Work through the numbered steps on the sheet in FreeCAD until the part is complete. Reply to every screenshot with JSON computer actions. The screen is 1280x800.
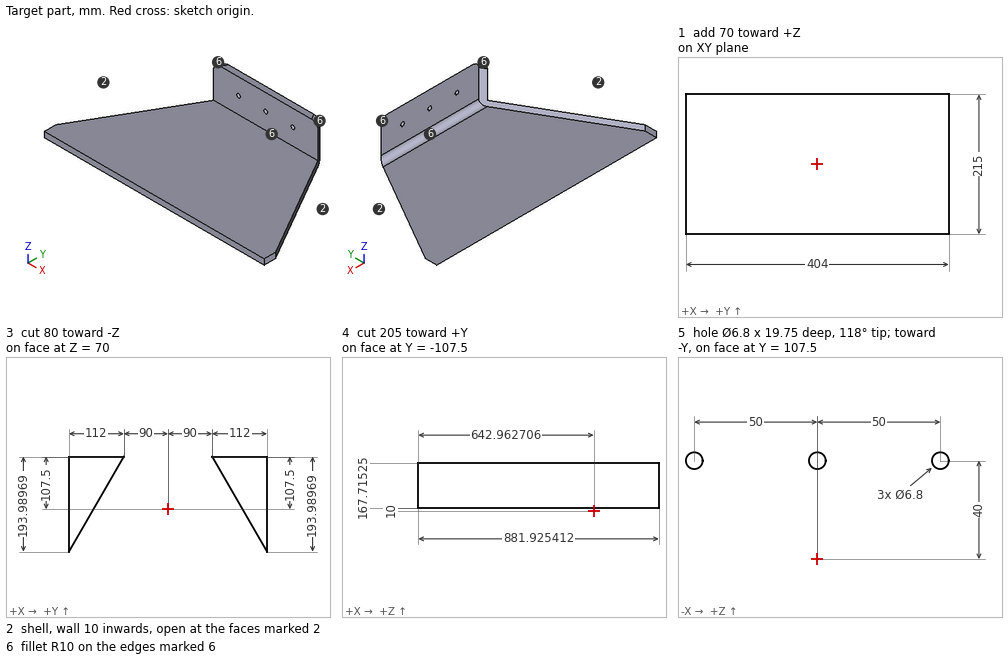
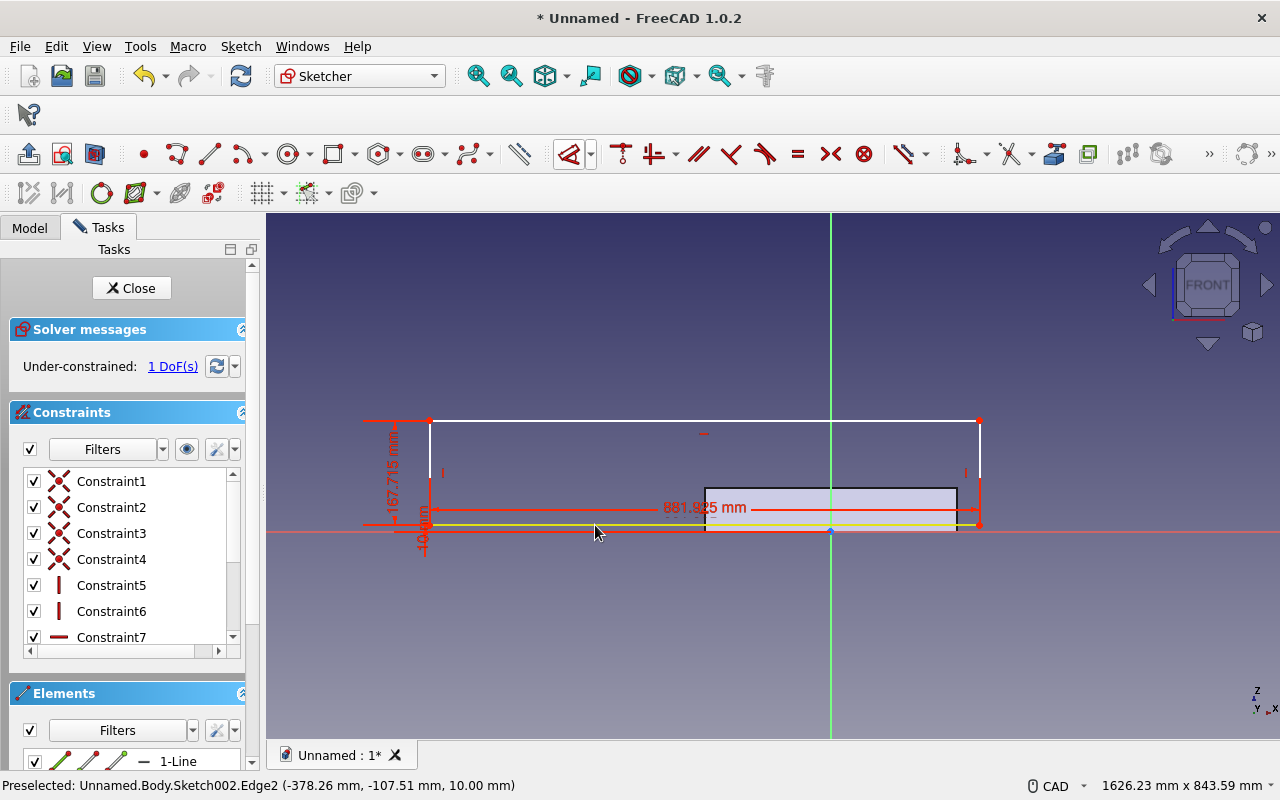
{"action": "left_click", "coordinate": [430, 421]}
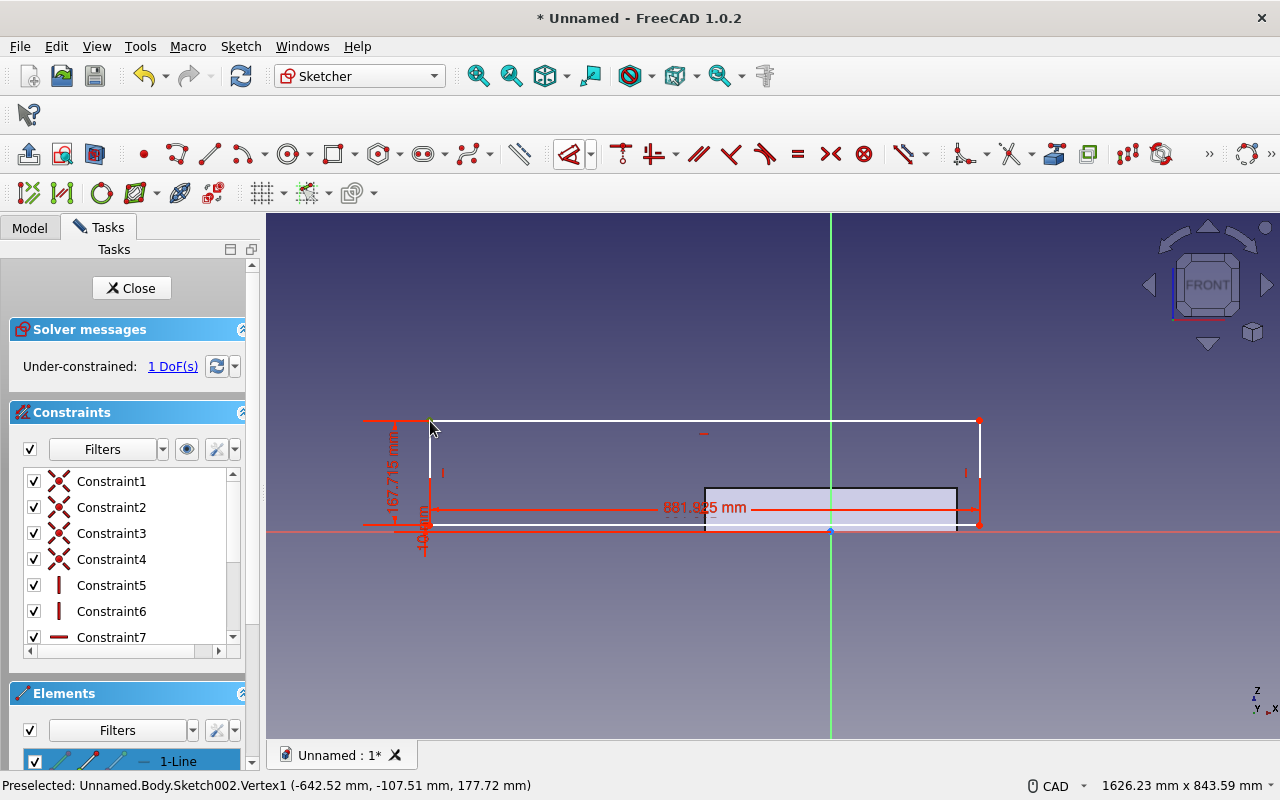
{"action": "left_click", "coordinate": [590, 154]}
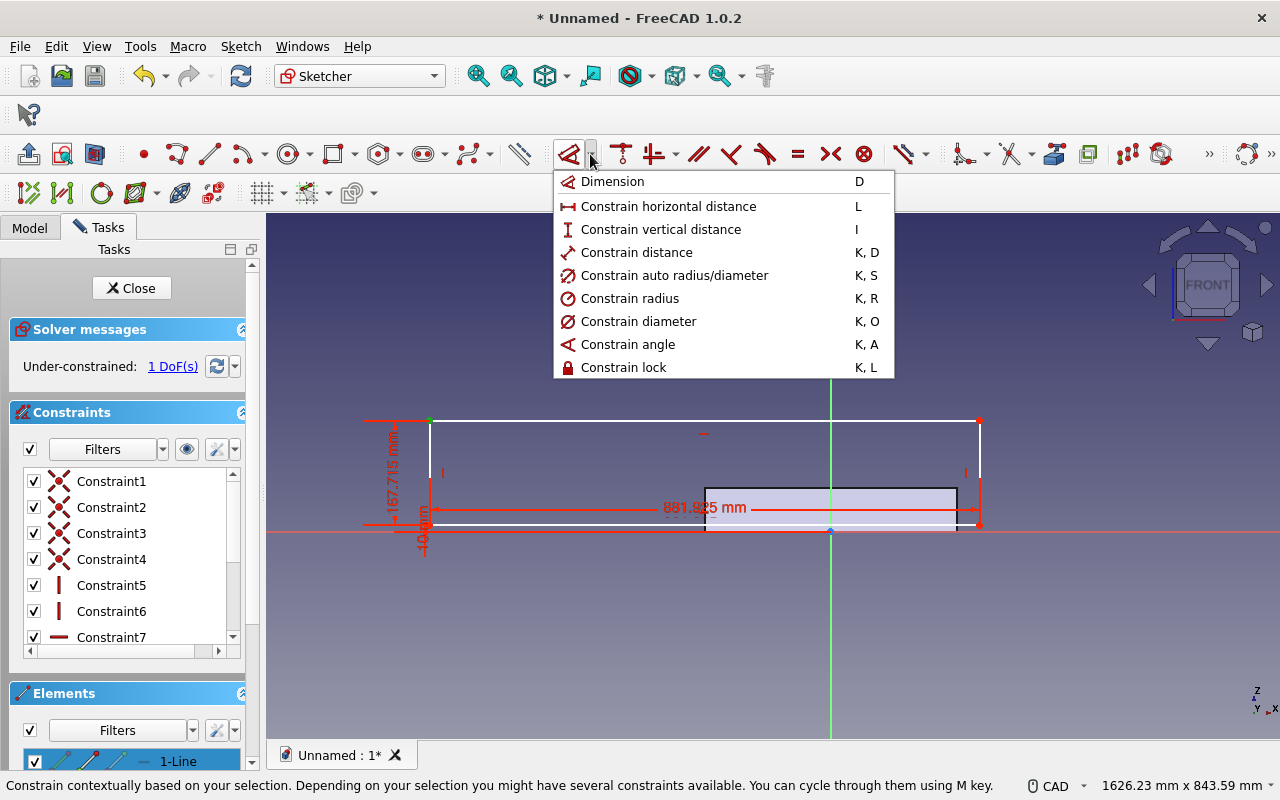
{"action": "left_click", "coordinate": [724, 206]}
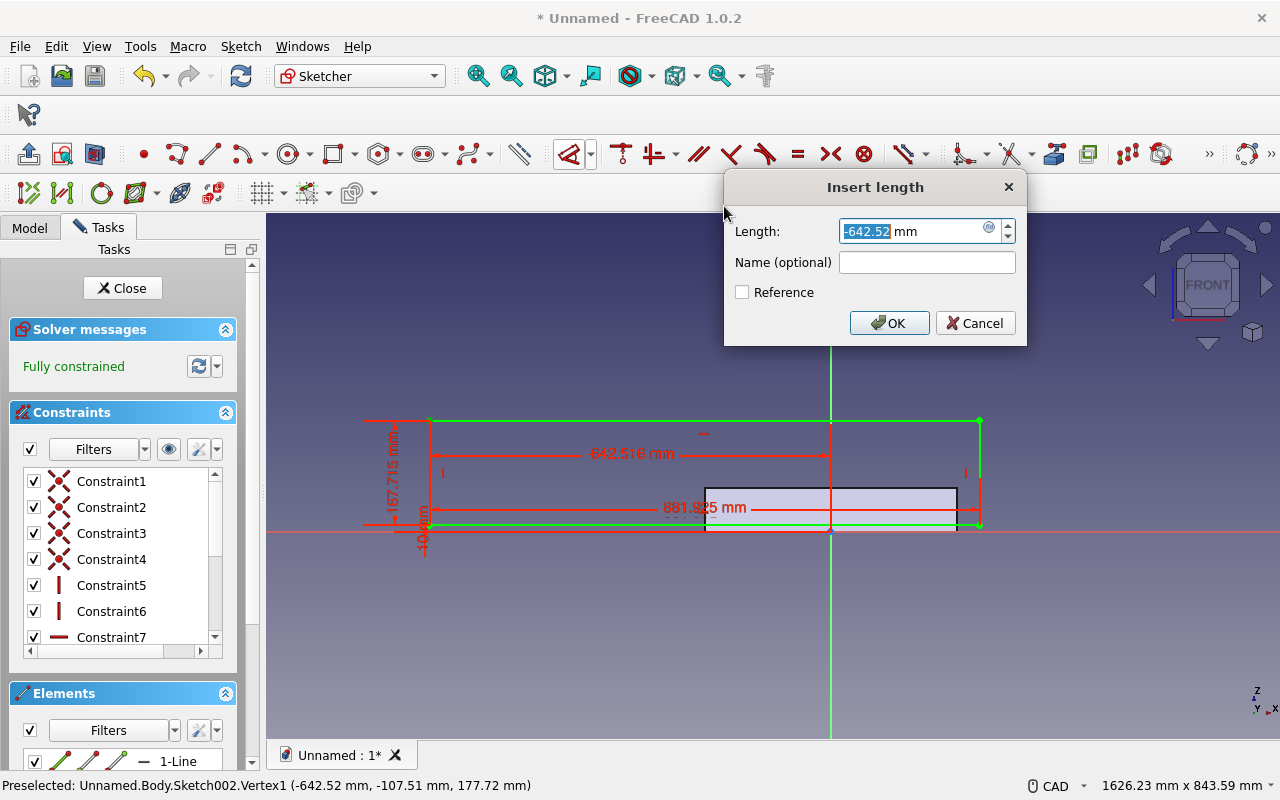
{"action": "type", "text": "-642.962706"}
{"action": "key", "text": "Return"}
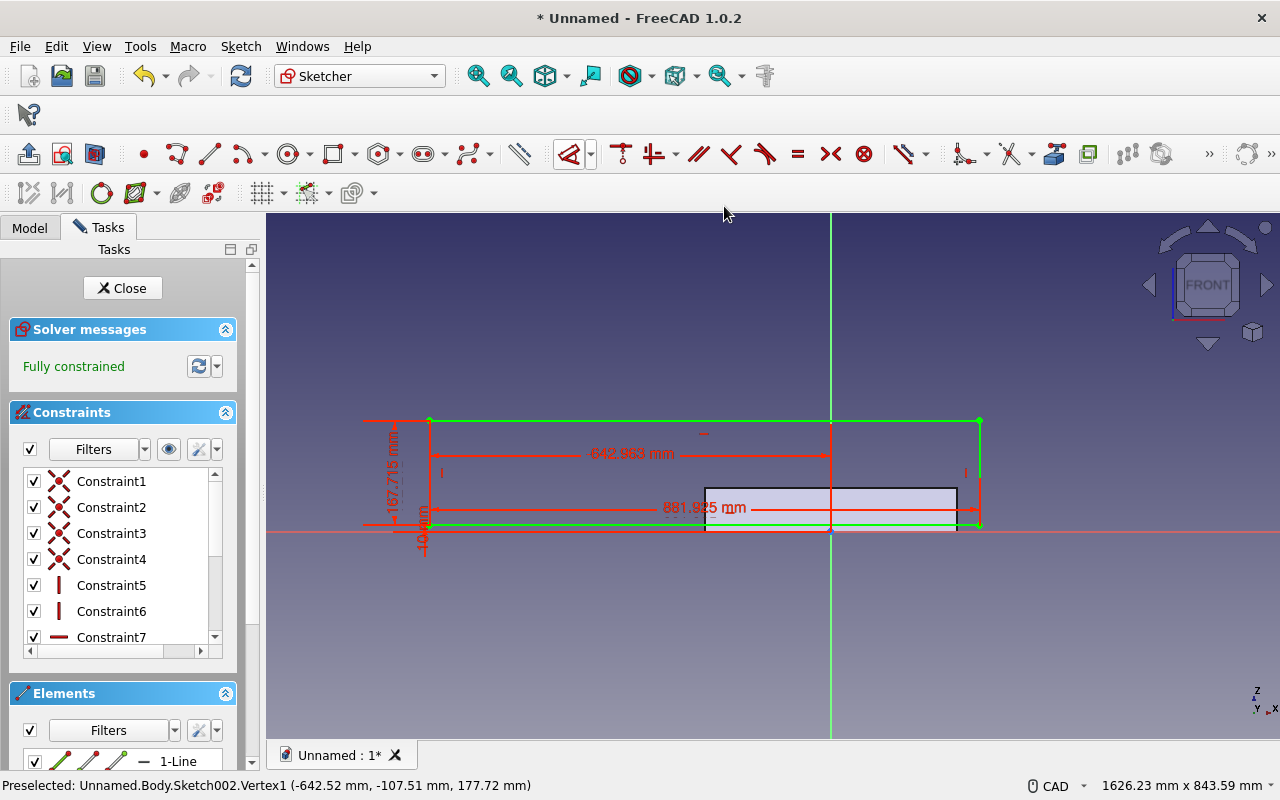
{"action": "left_click", "coordinate": [123, 288]}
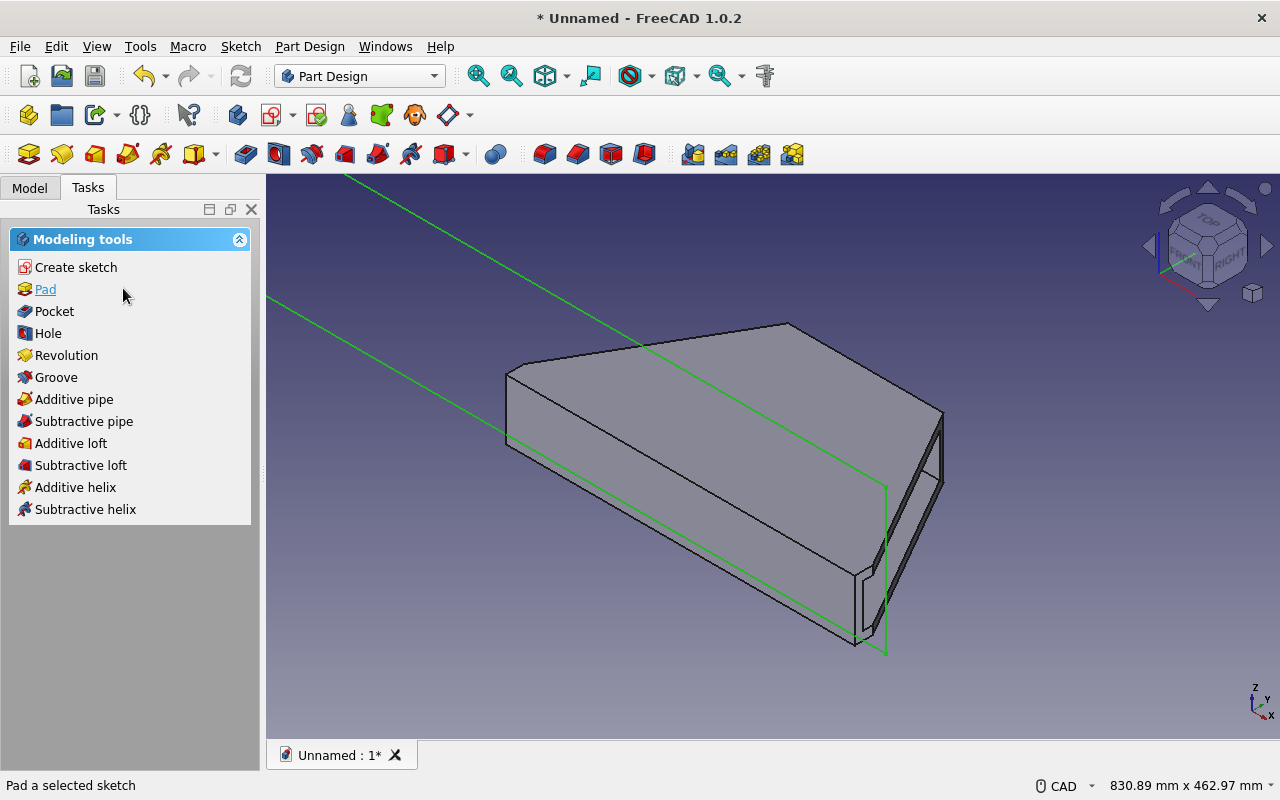
{"action": "left_click", "coordinate": [246, 154]}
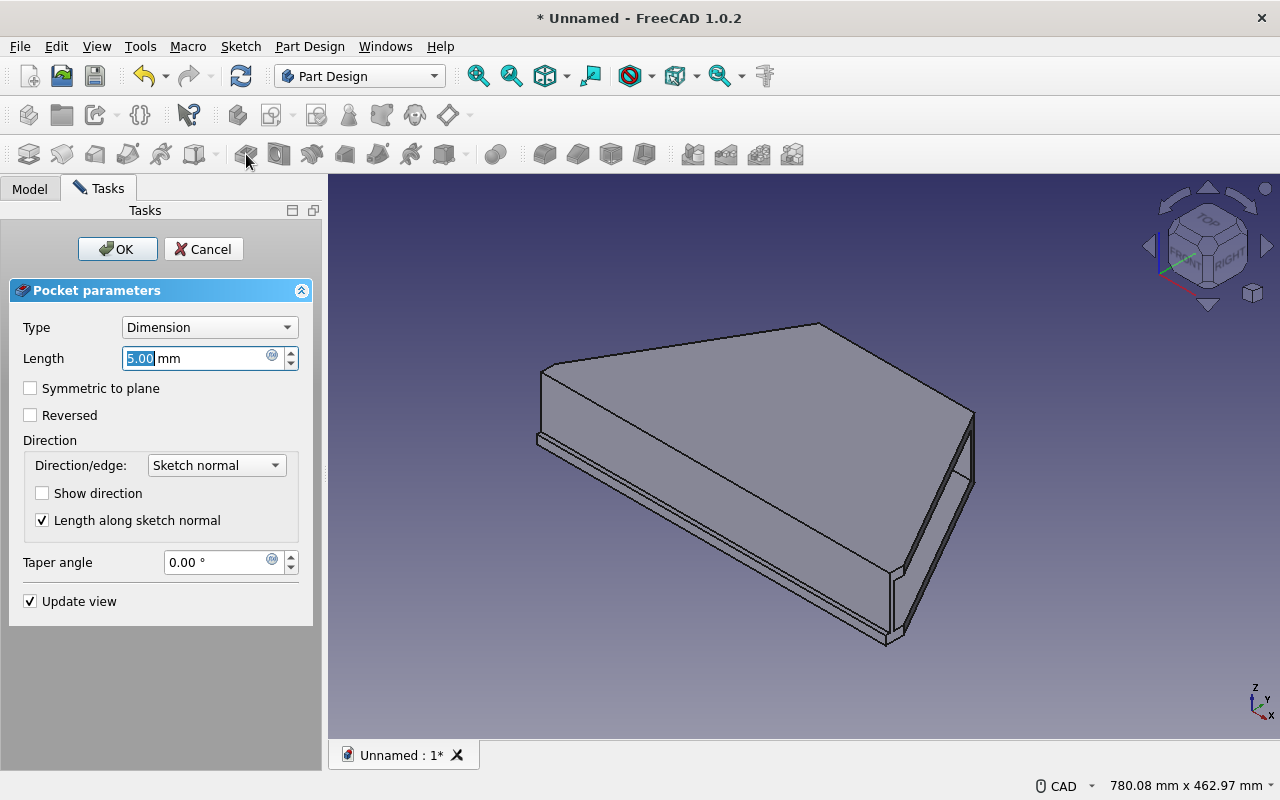
{"action": "type", "text": "205"}
{"action": "key", "text": "Tab"}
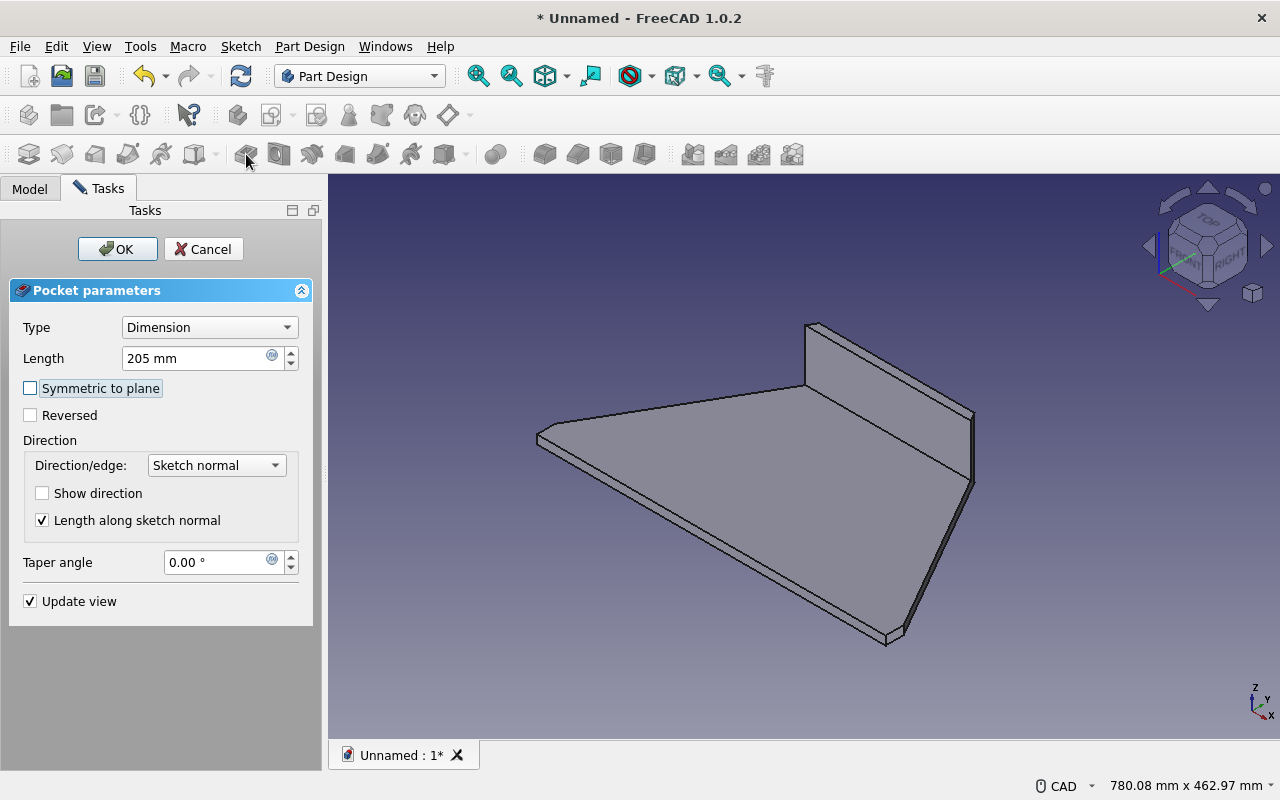
{"action": "left_click", "coordinate": [118, 249]}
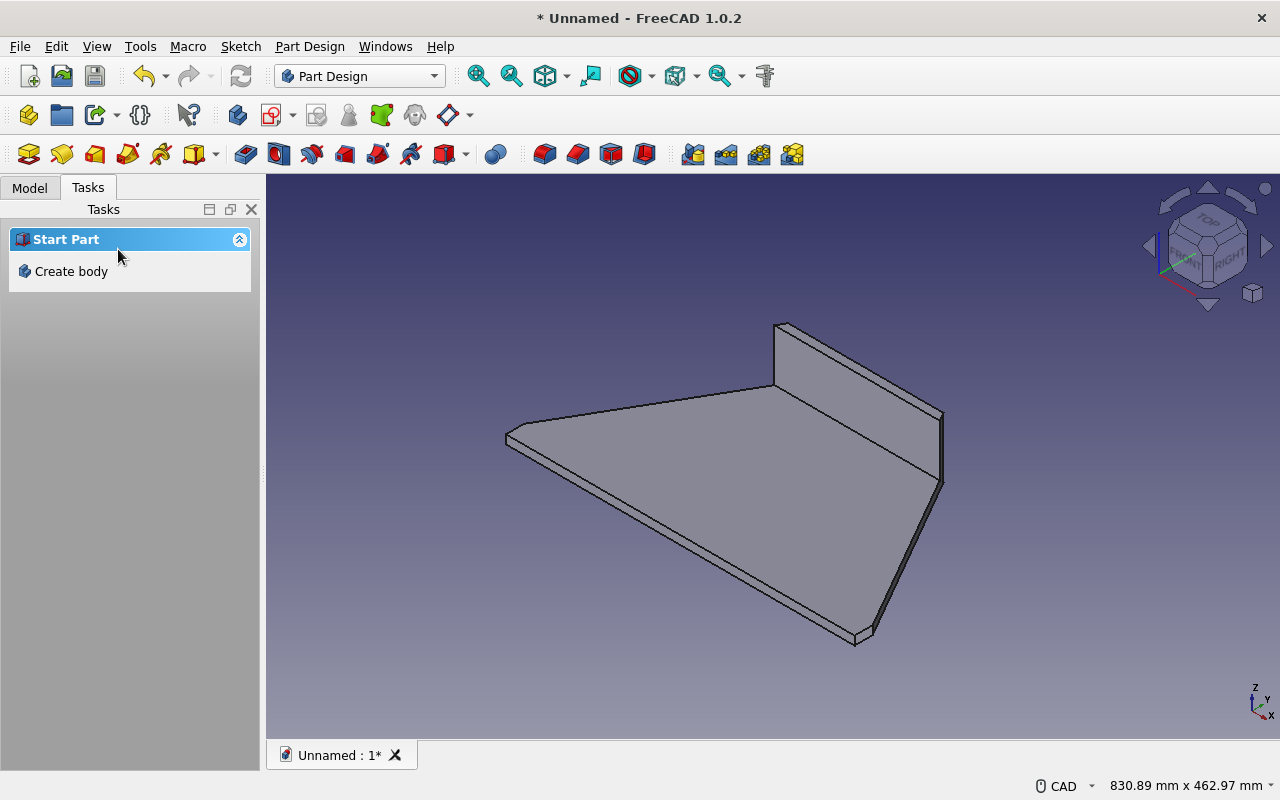
{"action": "key", "text": "4"}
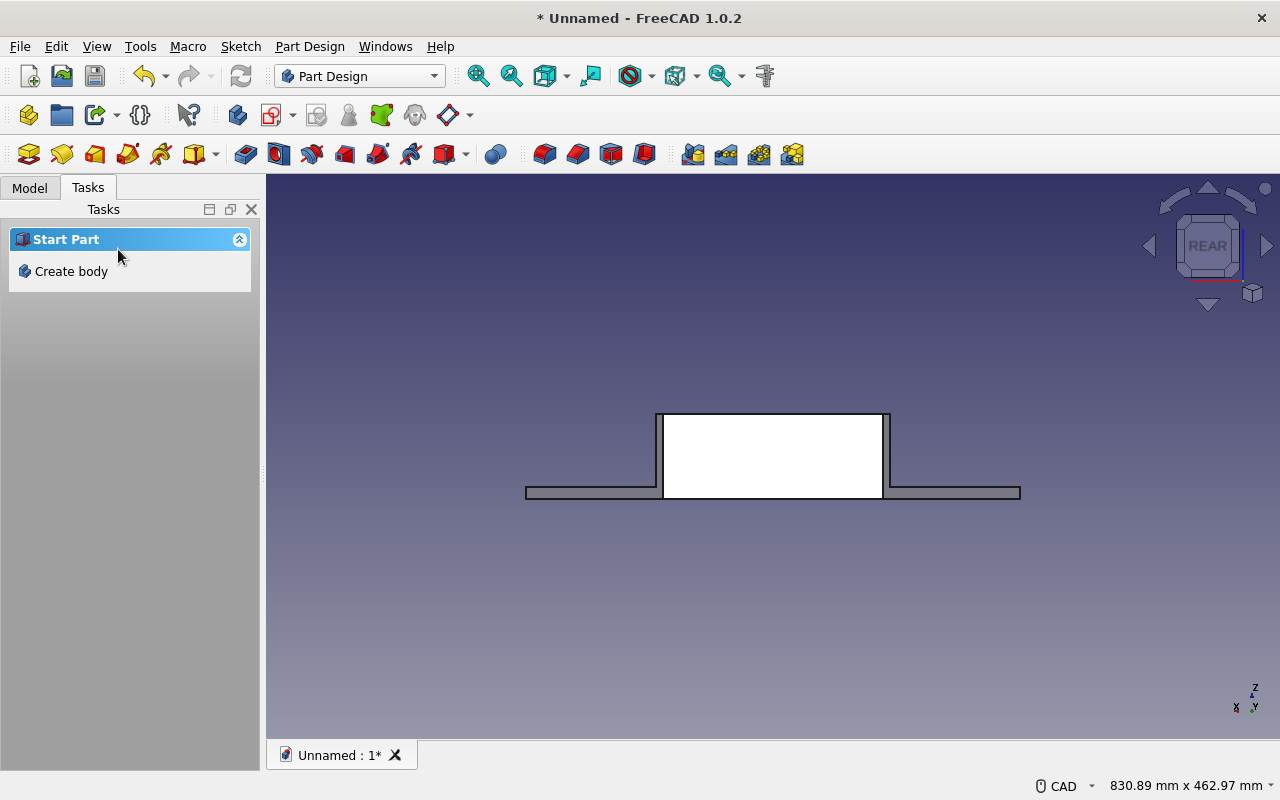
{"action": "left_click", "coordinate": [710, 456]}